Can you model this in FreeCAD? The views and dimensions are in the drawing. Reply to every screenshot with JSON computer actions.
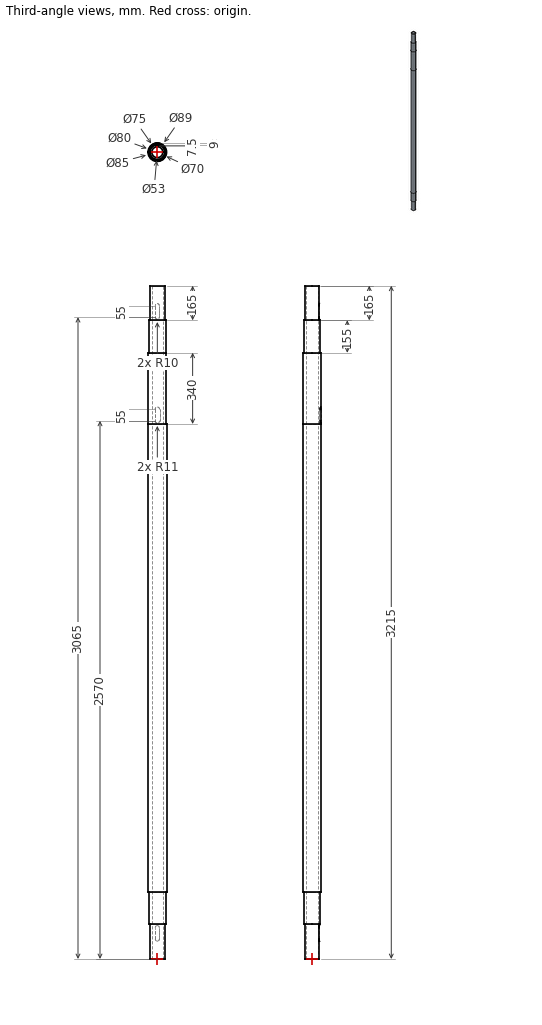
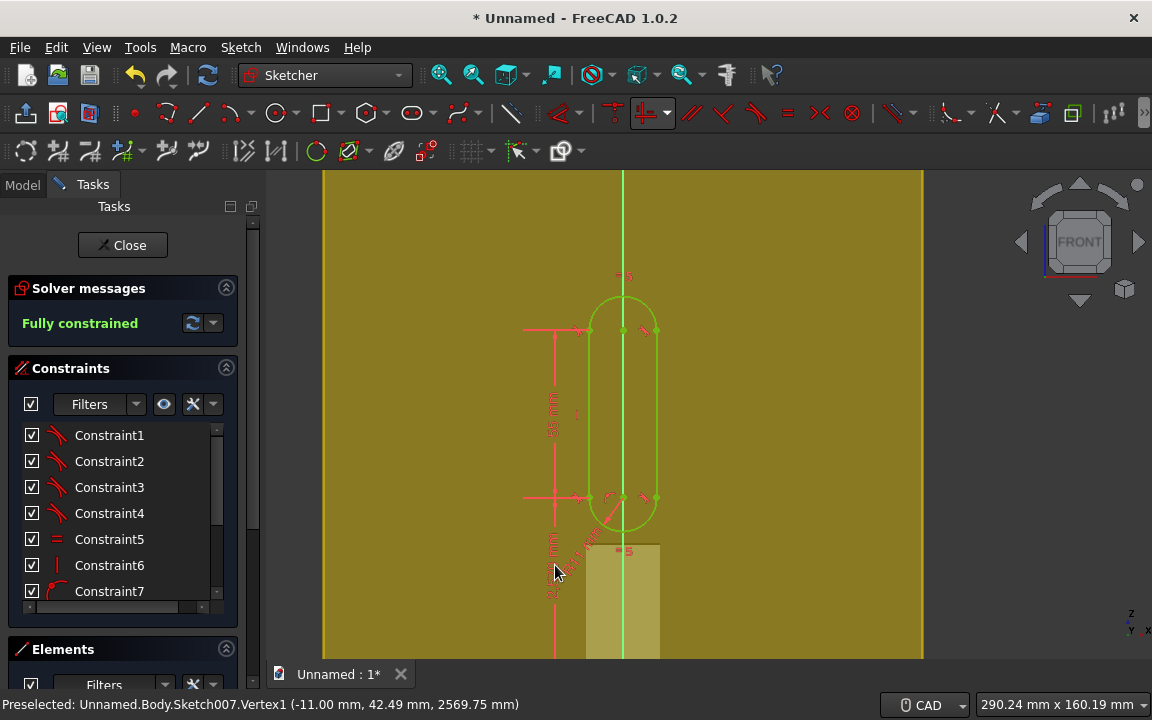
{"action": "left_click", "coordinate": [123, 245]}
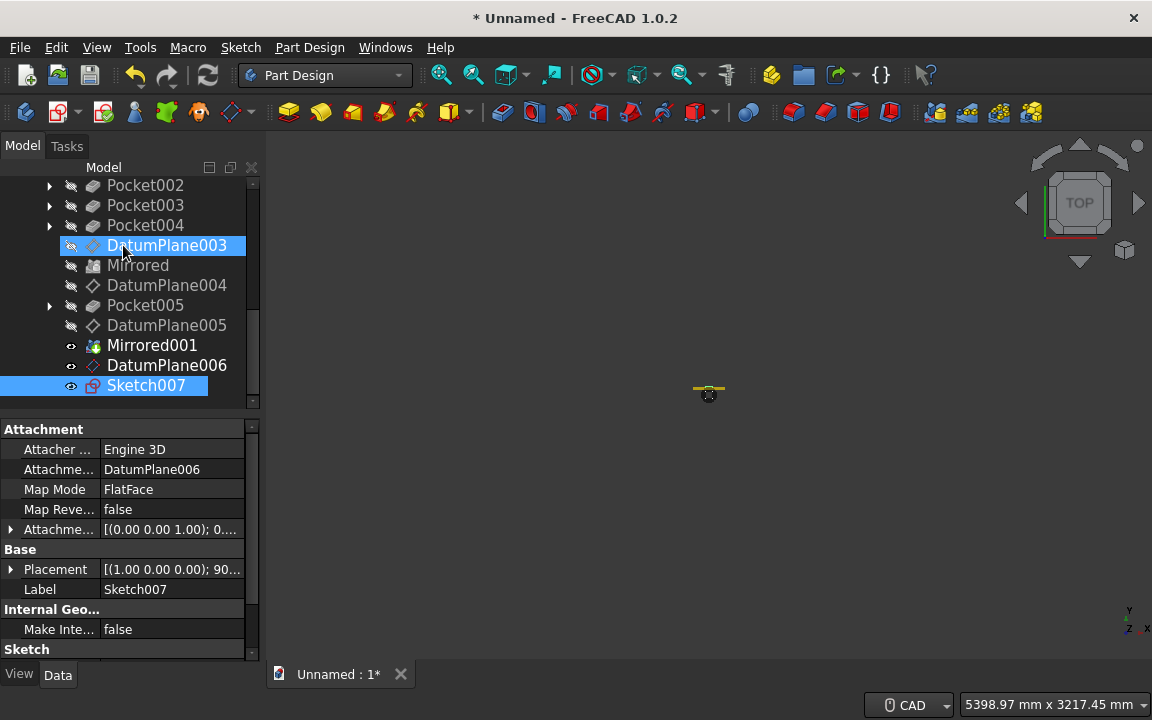
{"action": "left_click", "coordinate": [504, 112]}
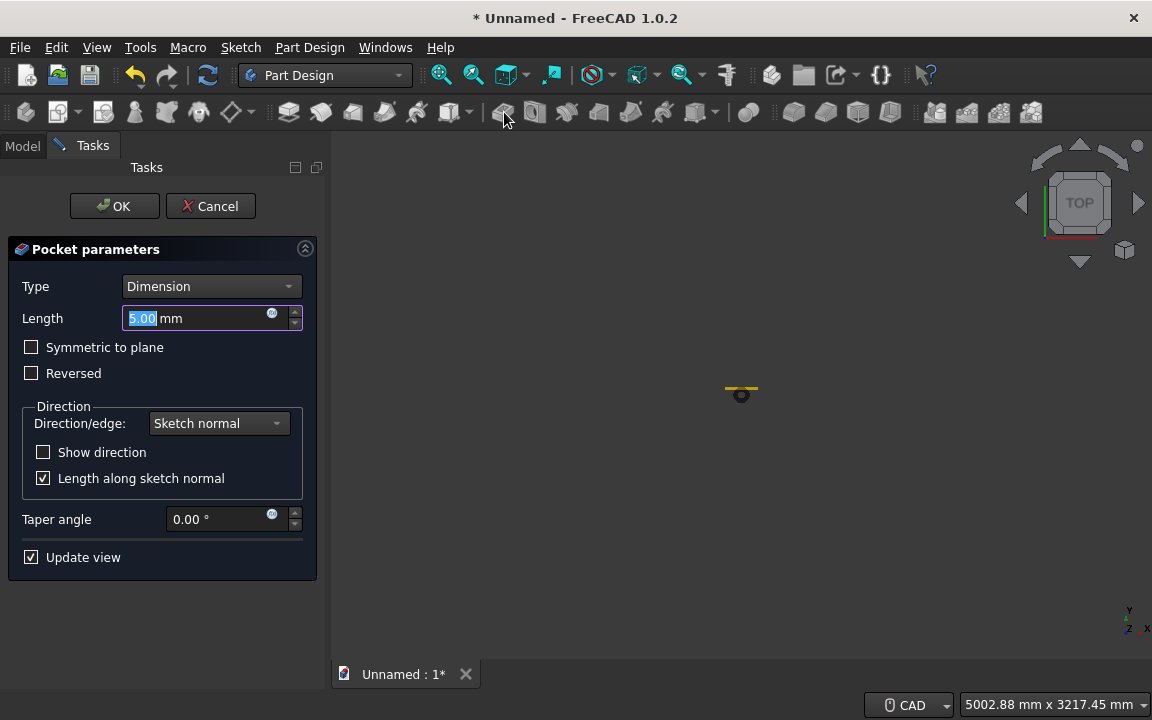
{"action": "type", "text": "9"}
{"action": "key", "text": "Tab"}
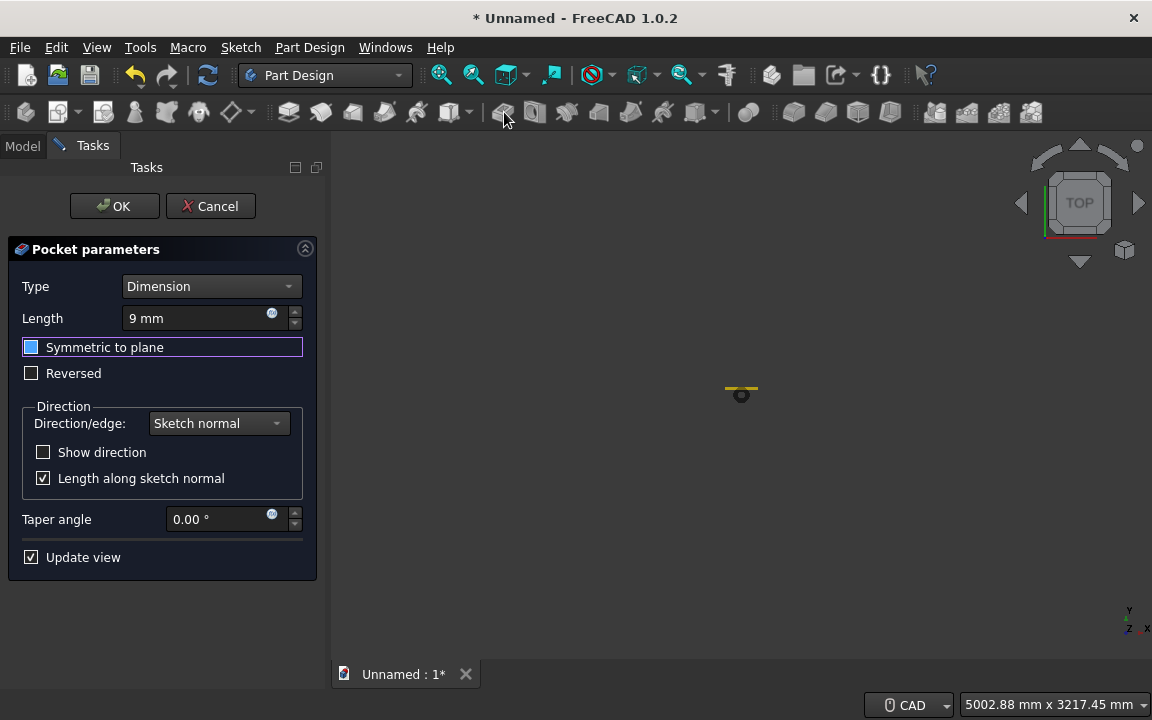
{"action": "left_click", "coordinate": [30, 373]}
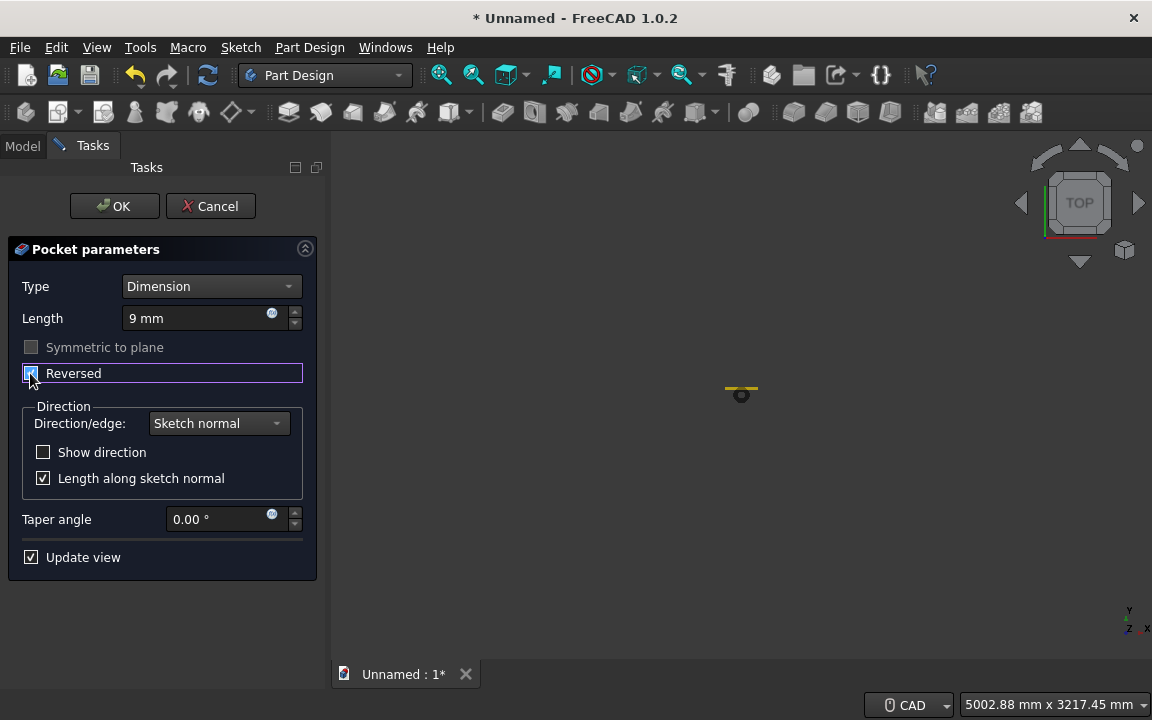
{"action": "left_click", "coordinate": [115, 206]}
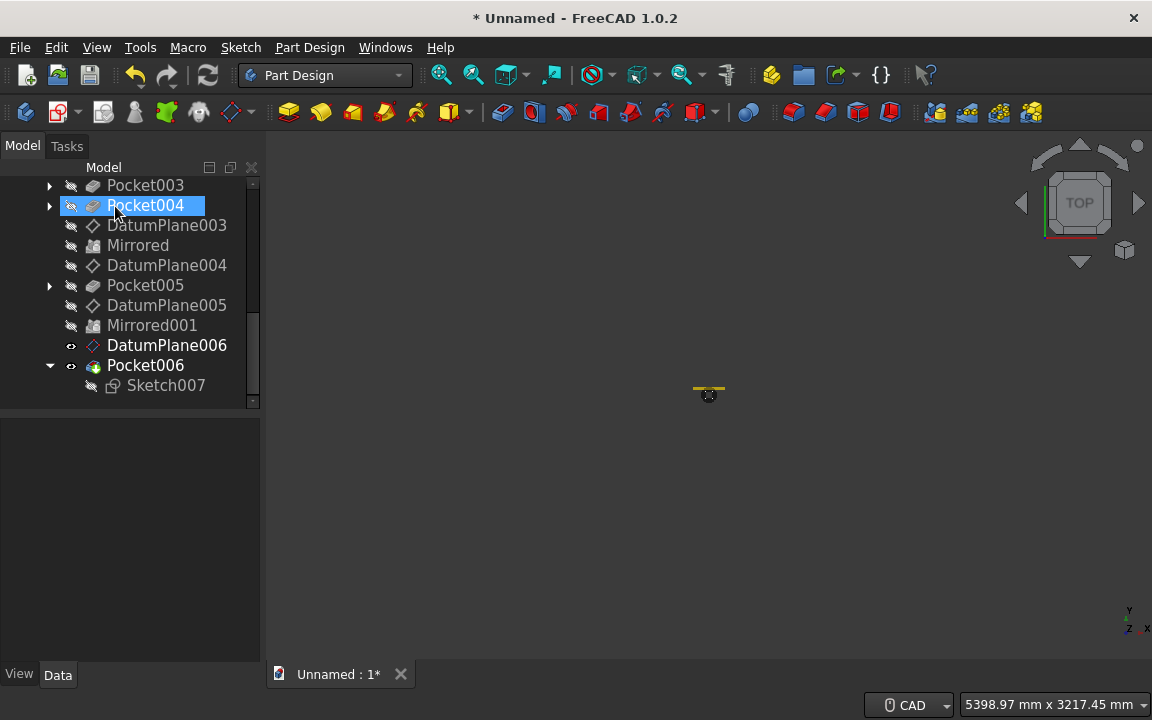
{"action": "left_click", "coordinate": [116, 346]}
{"action": "key", "text": "space"}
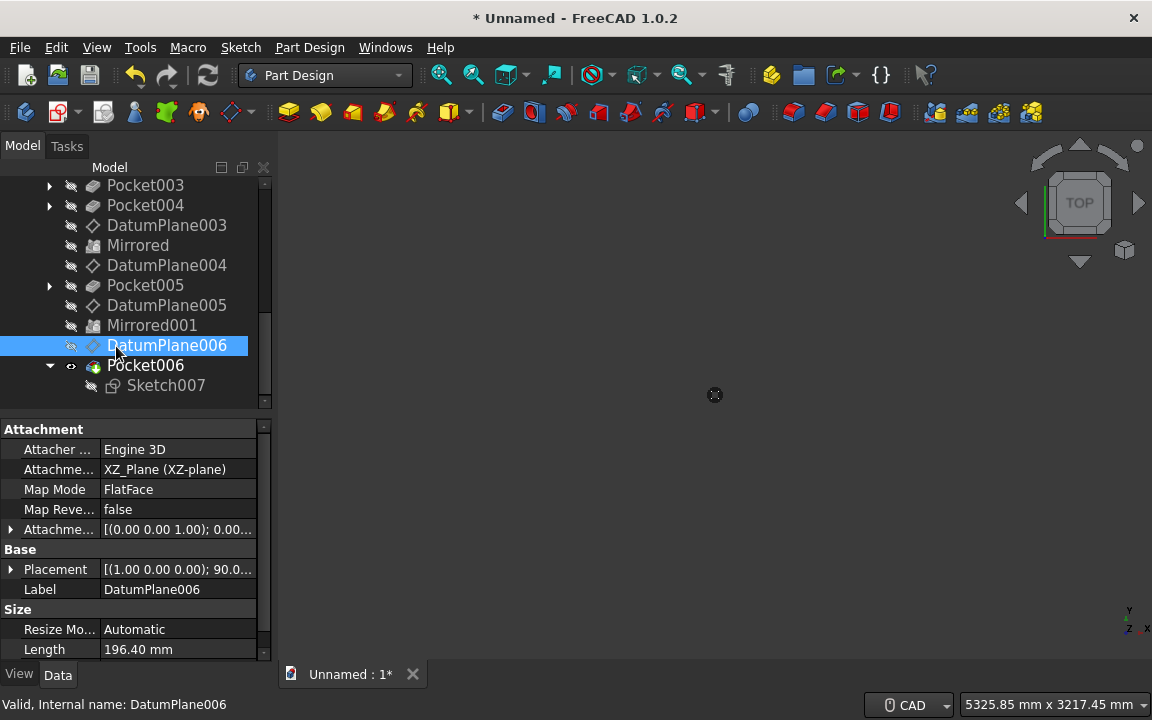
{"action": "key", "text": "0"}